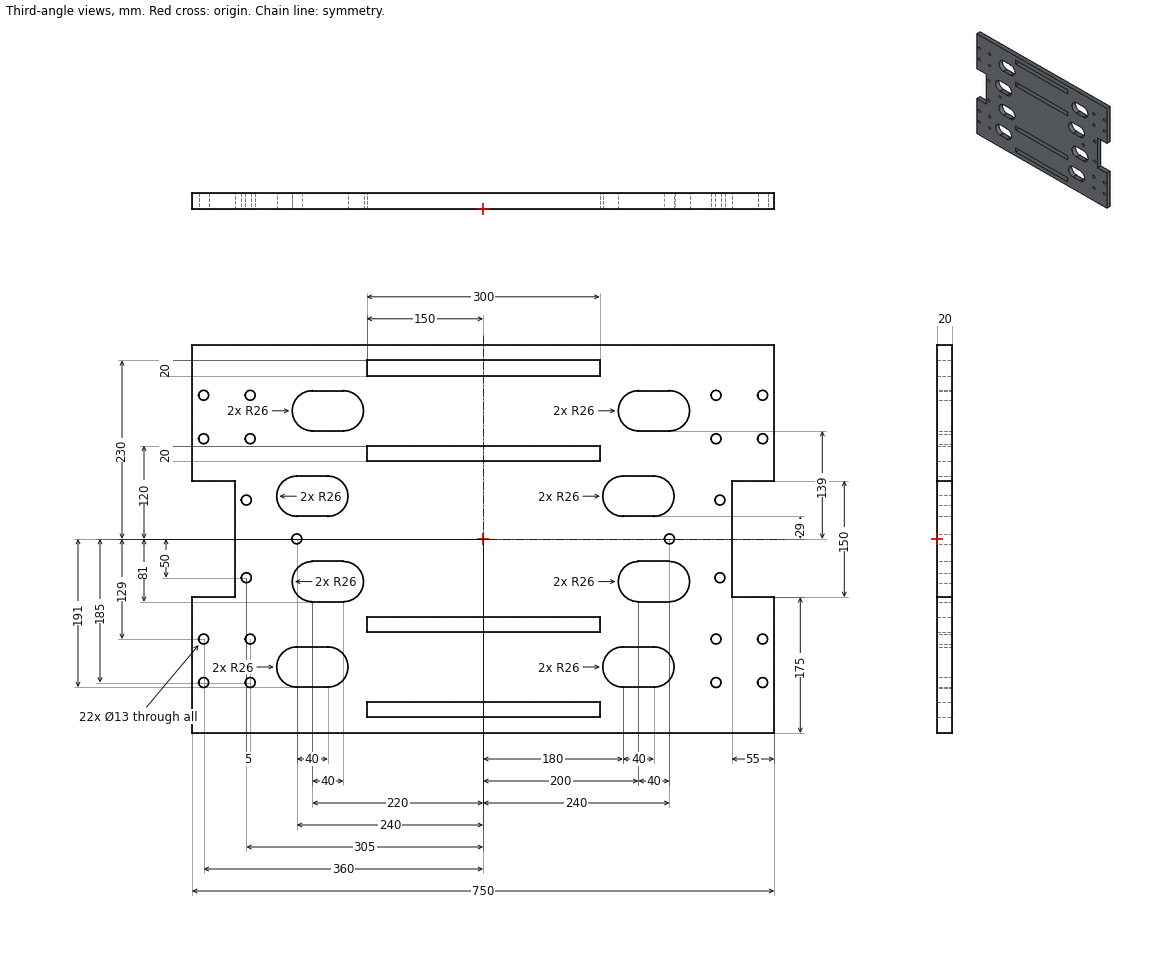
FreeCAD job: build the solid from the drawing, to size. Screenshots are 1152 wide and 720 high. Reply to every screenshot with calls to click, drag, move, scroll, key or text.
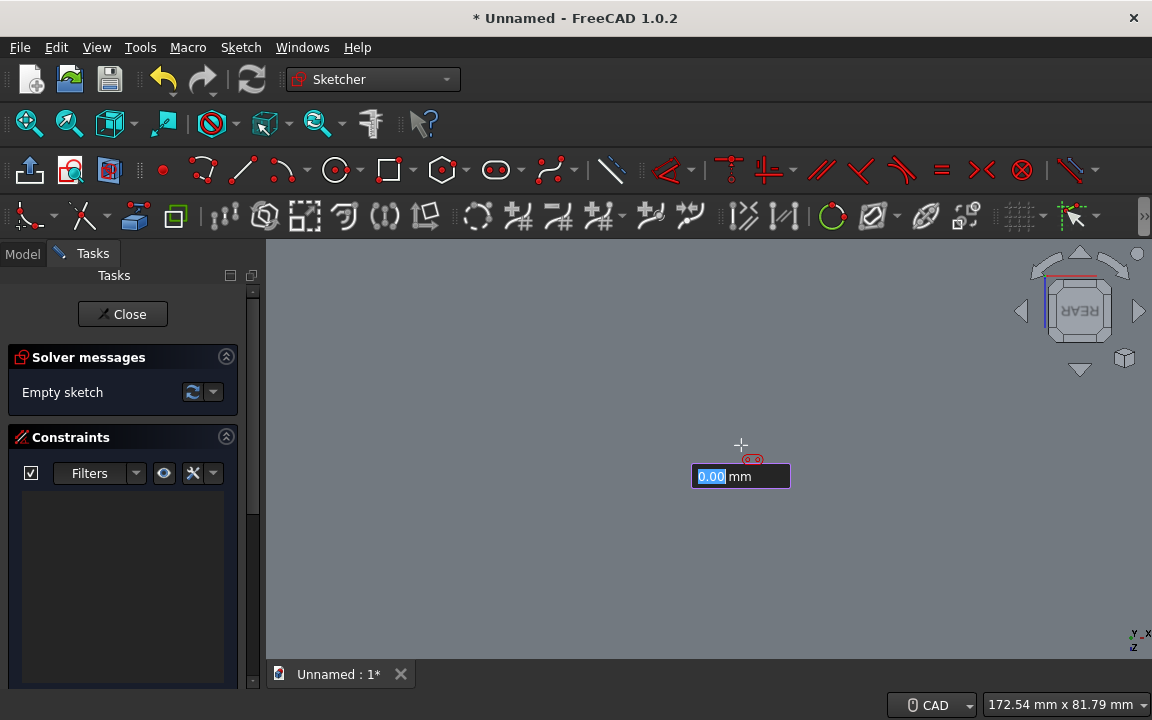
click(638, 312)
key(Escape)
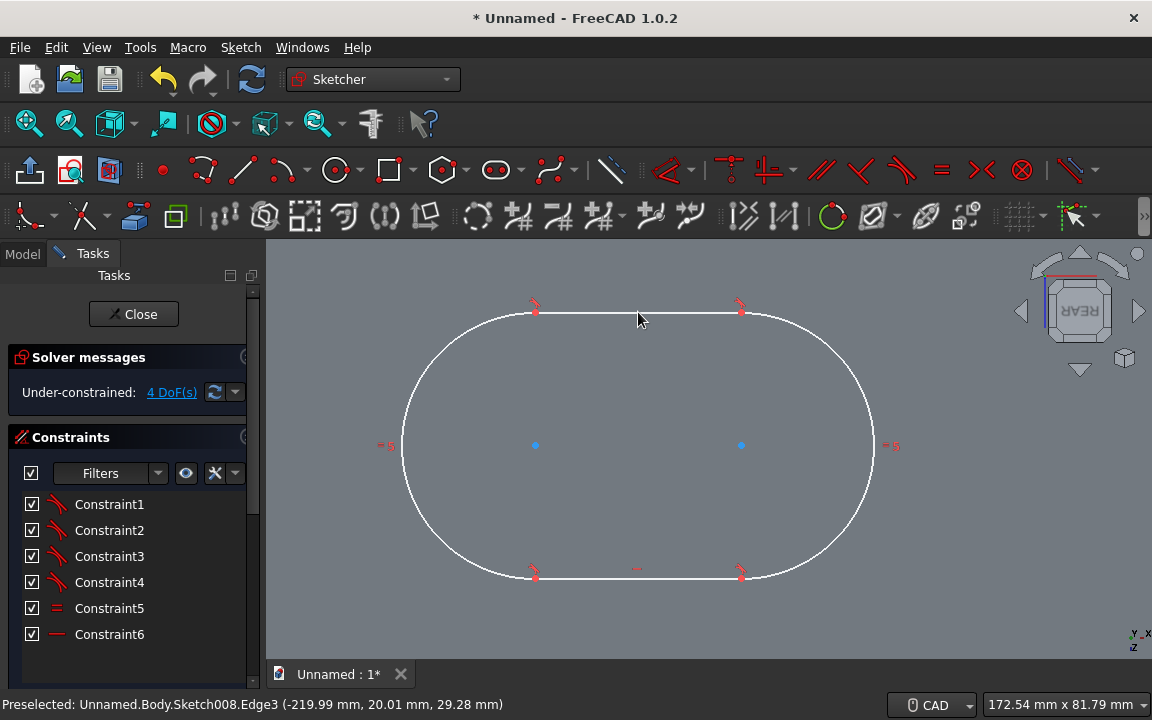
click(666, 170)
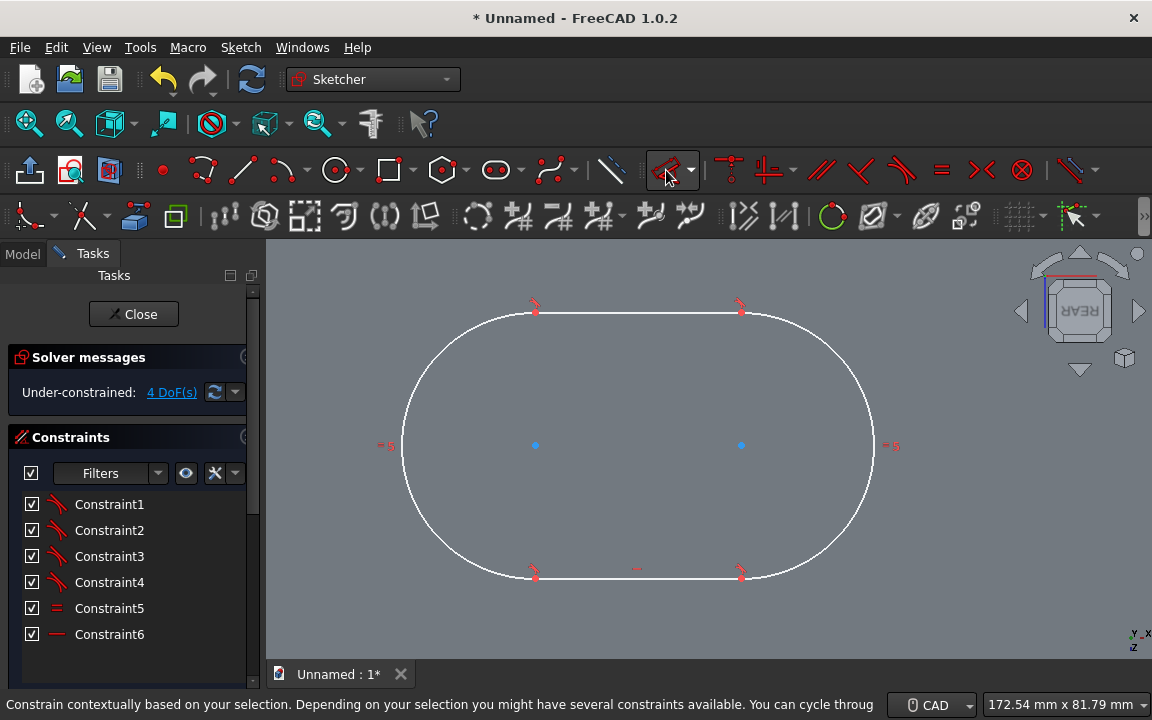
click(427, 368)
click(401, 349)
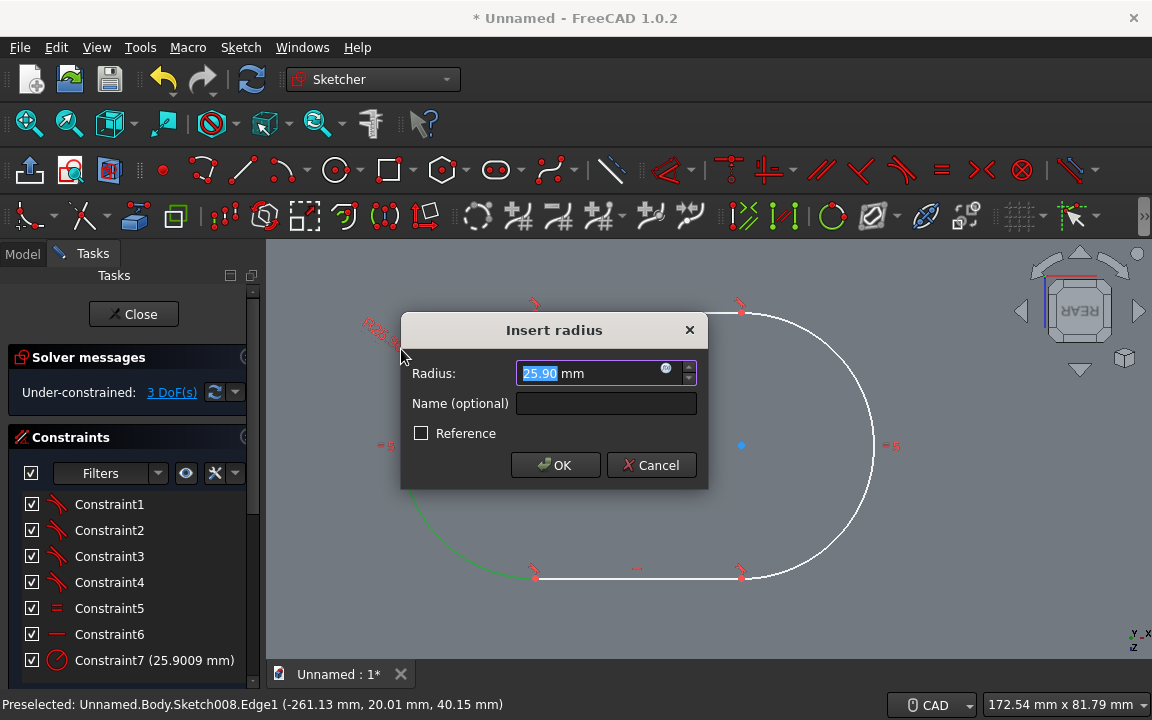
text(26)
key(Return)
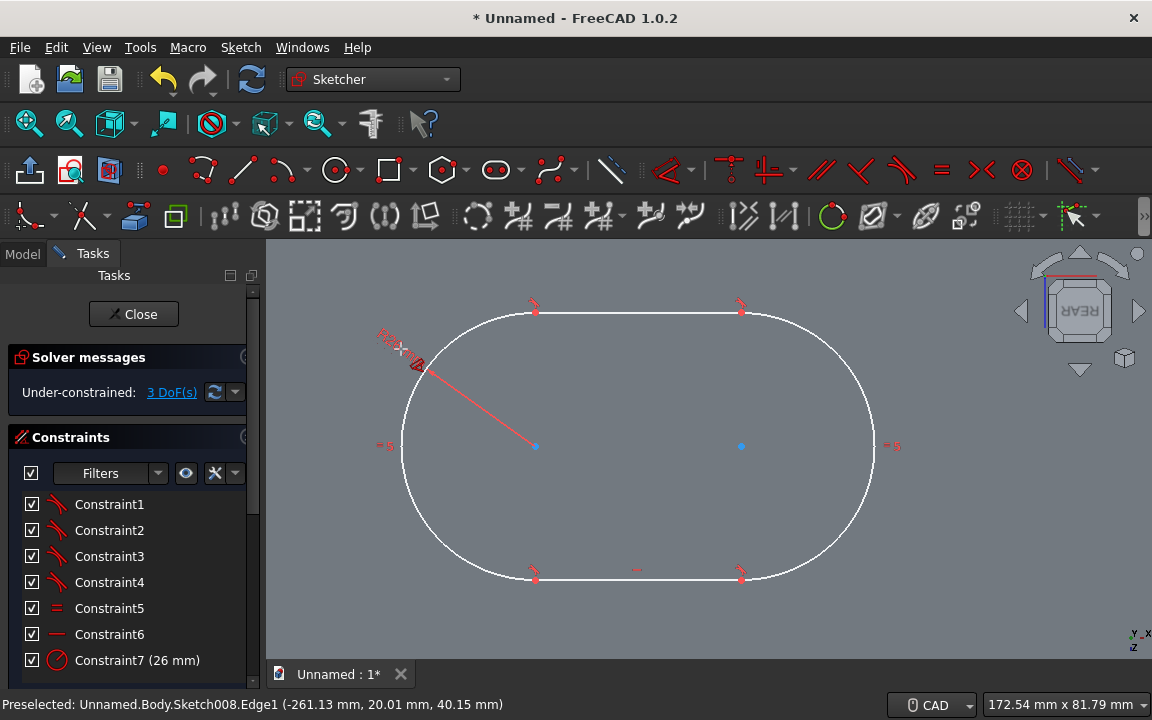
click(597, 313)
click(638, 279)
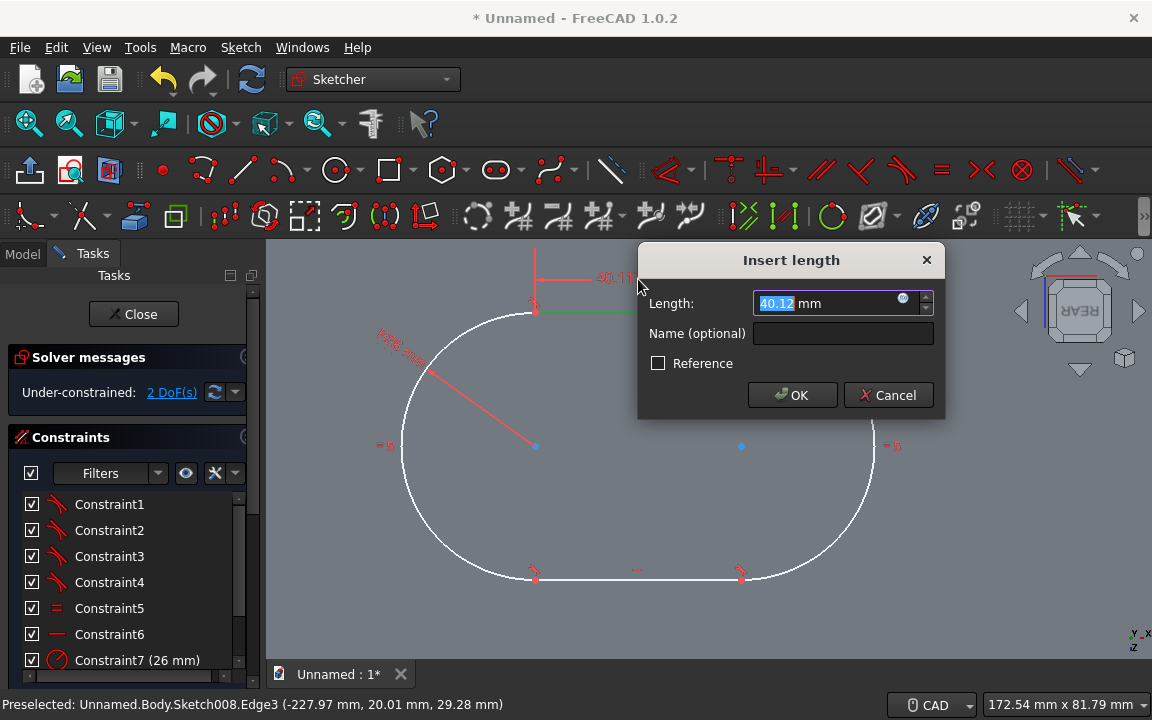
text(40)
key(Return)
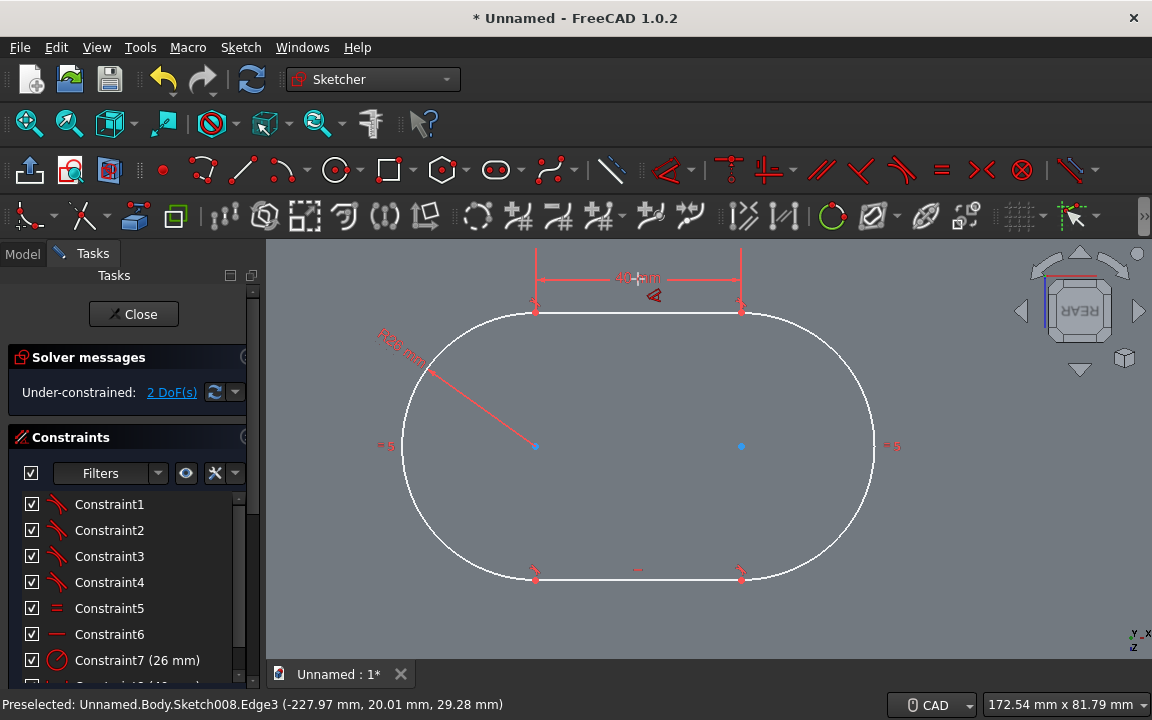
click(536, 313)
click(502, 290)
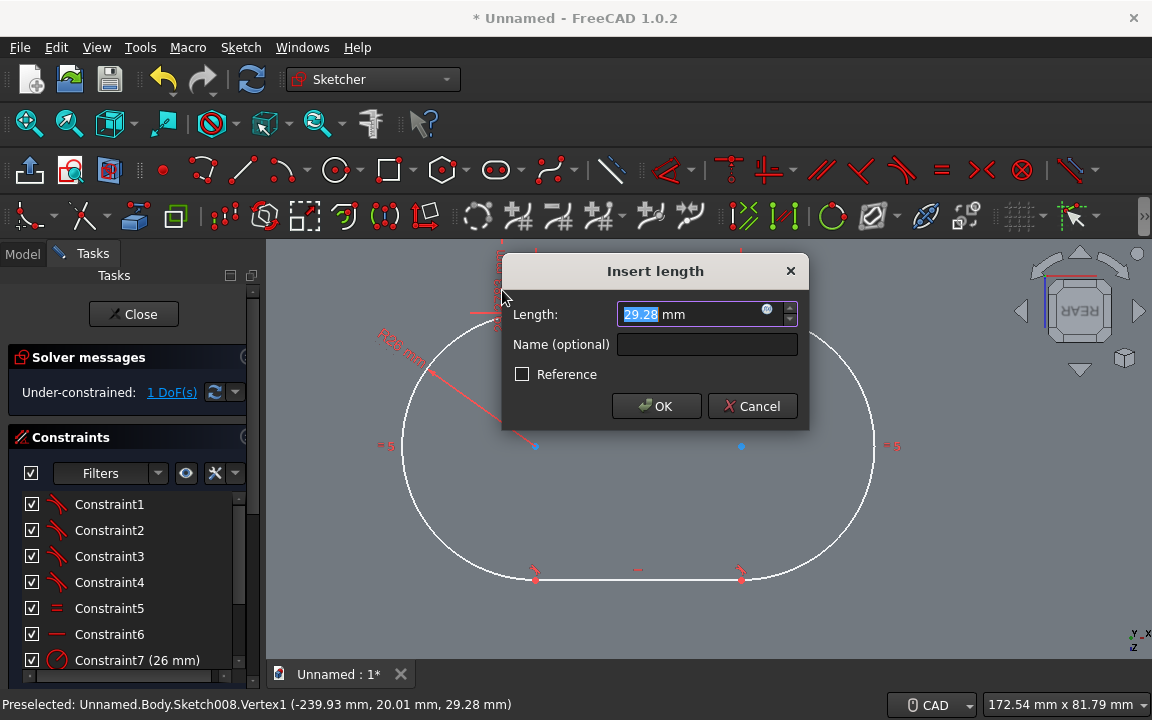
text(29)
key(Return)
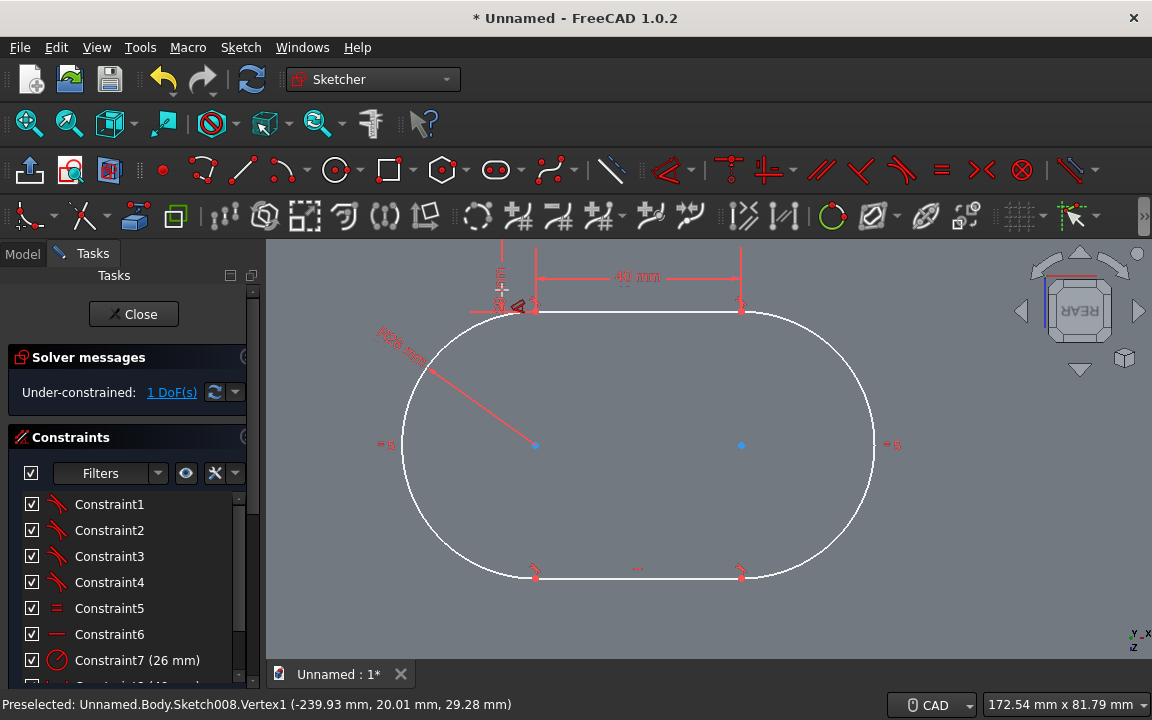
click(536, 312)
click(761, 346)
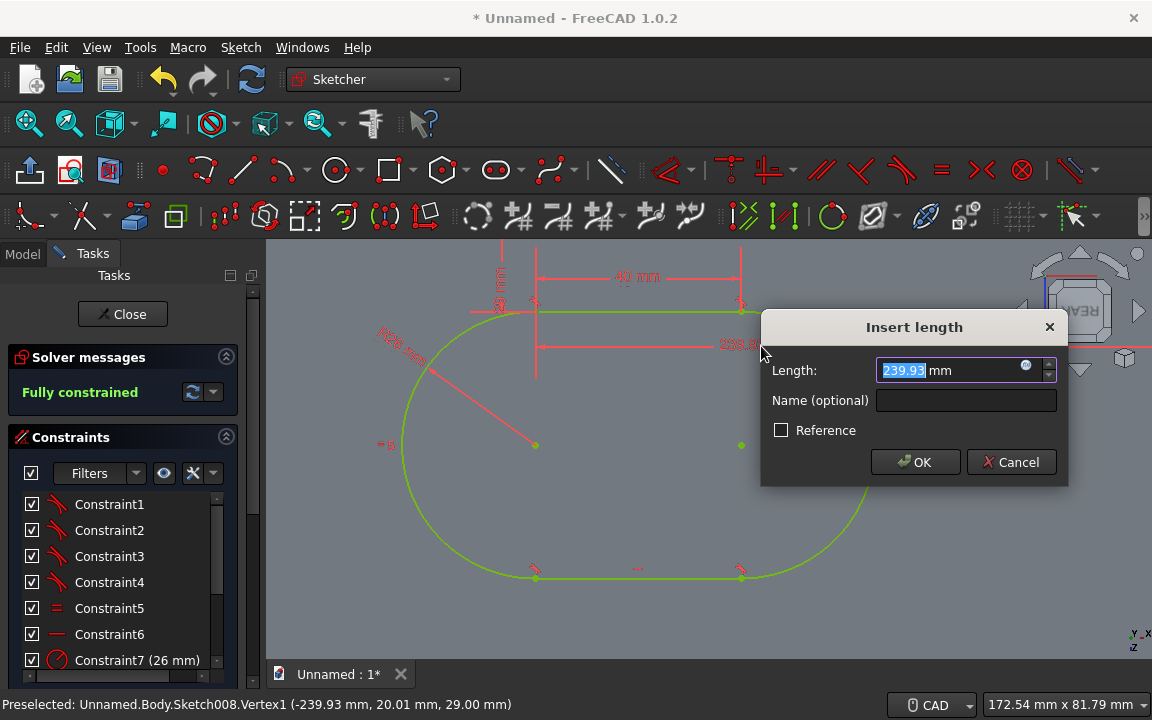
text(240)
key(Return)
key(Escape)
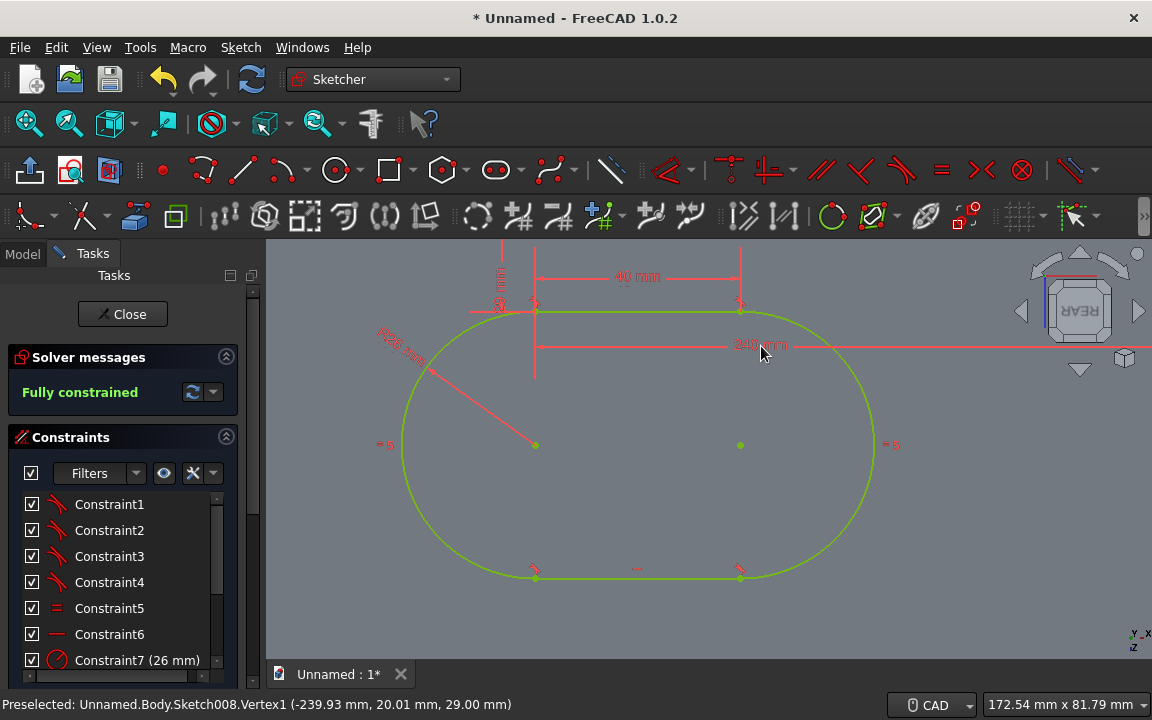
click(123, 314)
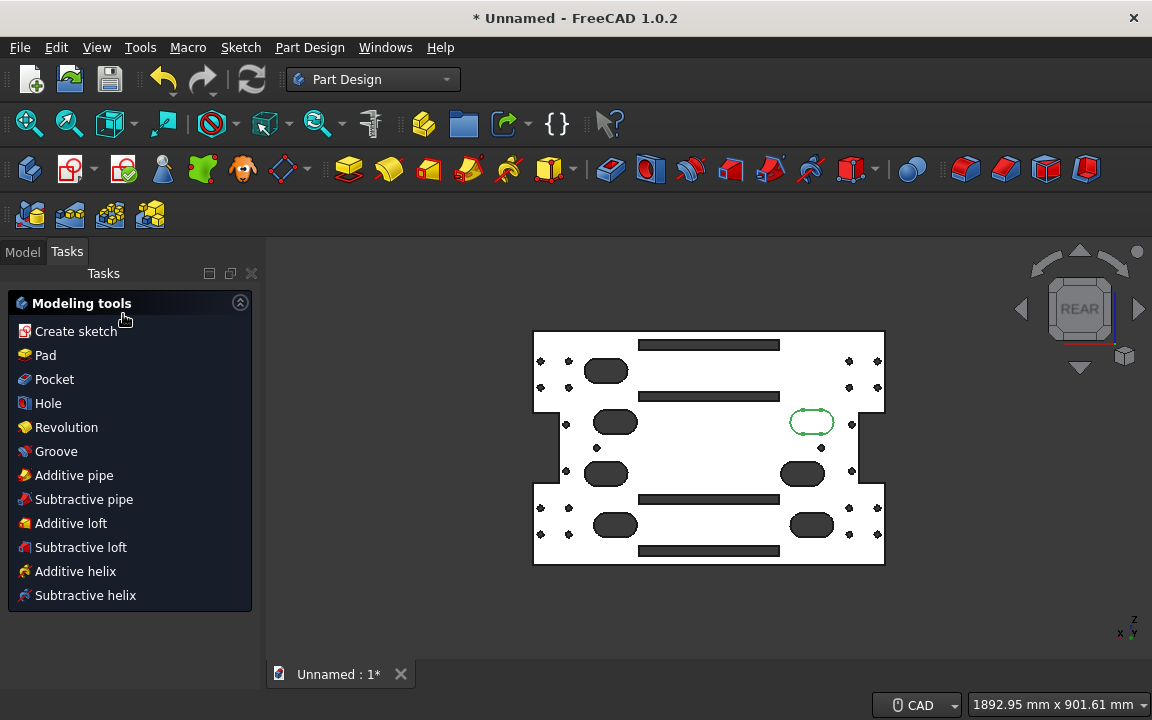
click(612, 170)